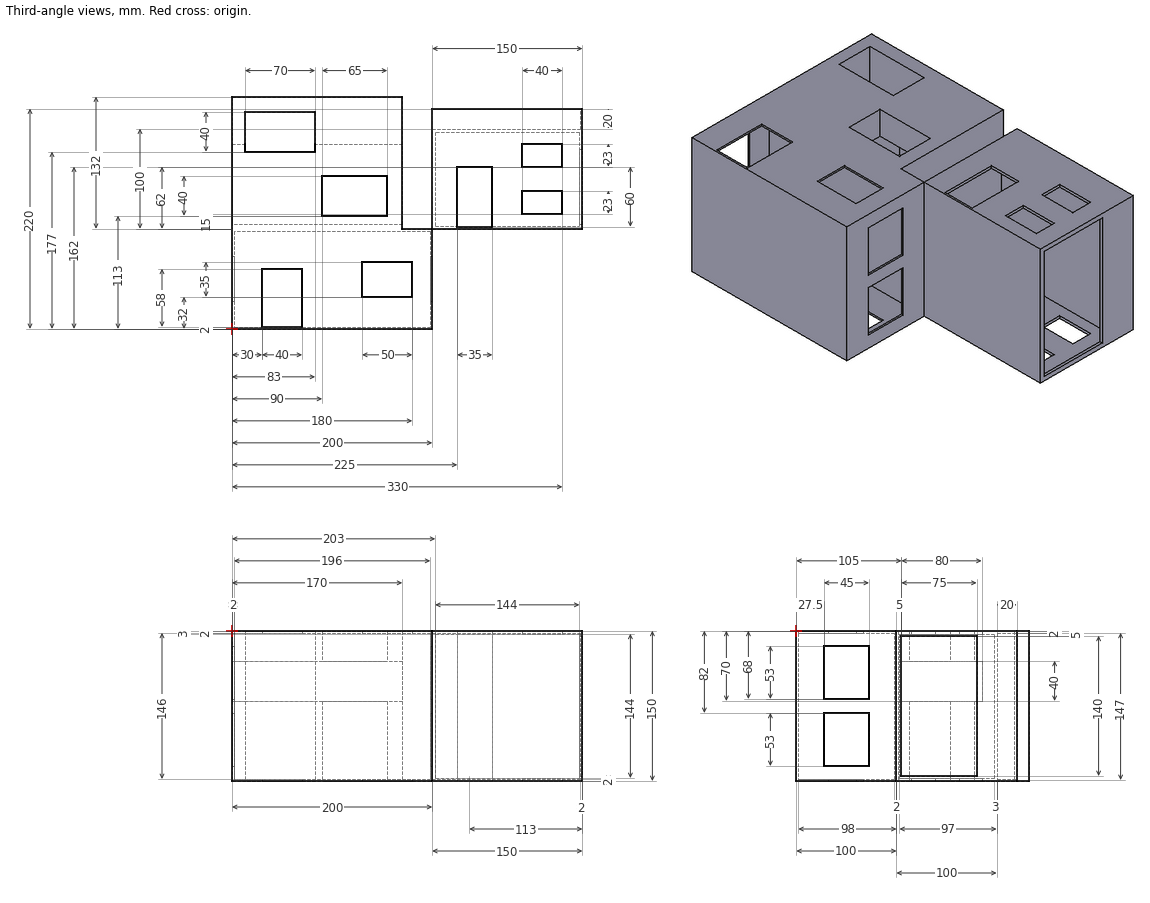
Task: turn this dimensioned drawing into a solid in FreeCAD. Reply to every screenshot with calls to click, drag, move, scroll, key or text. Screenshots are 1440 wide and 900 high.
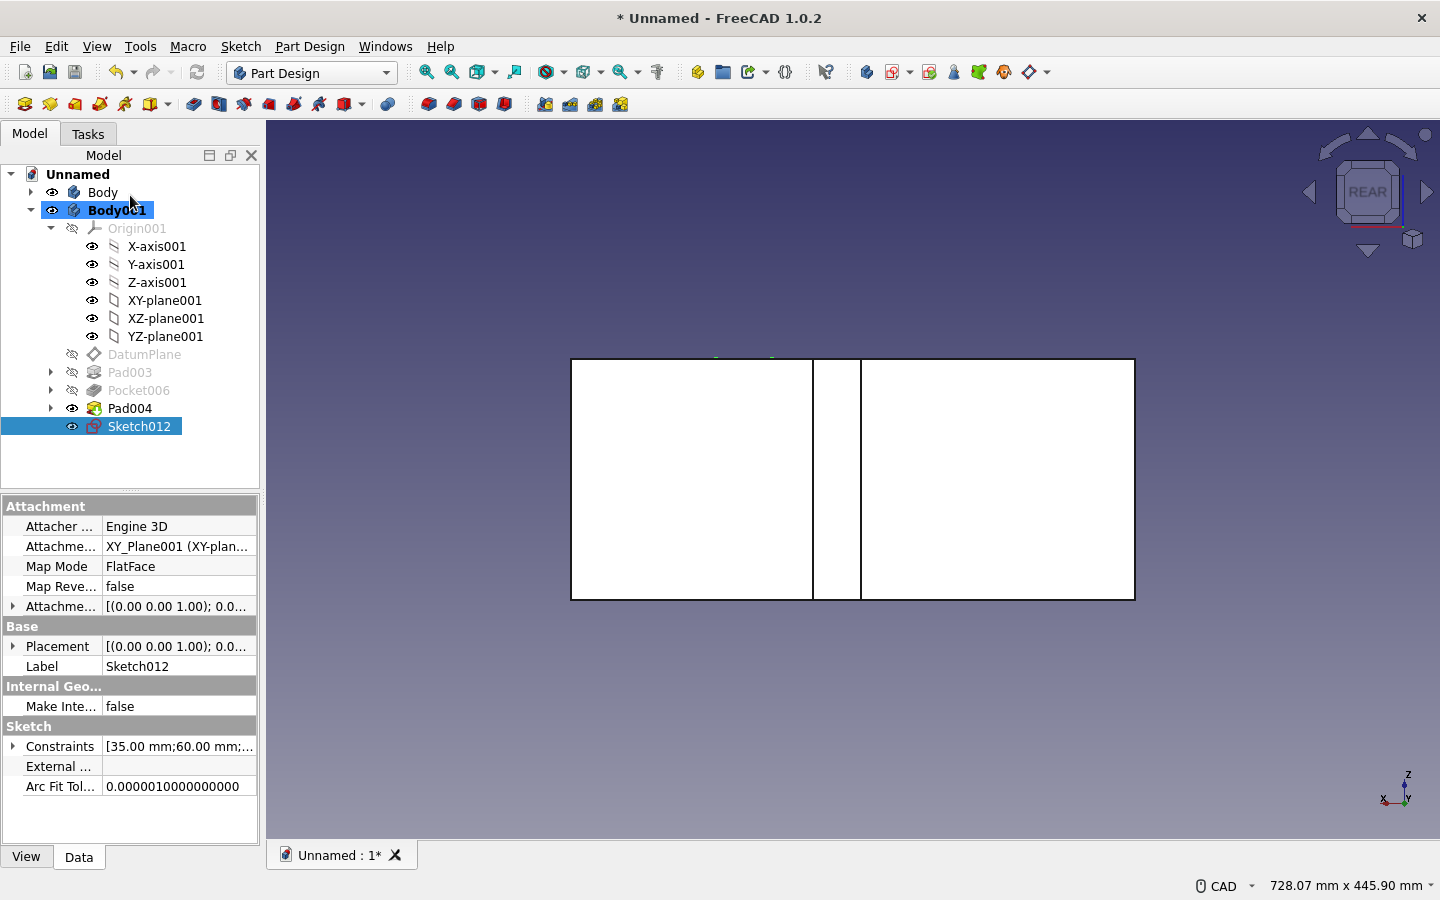
click(194, 104)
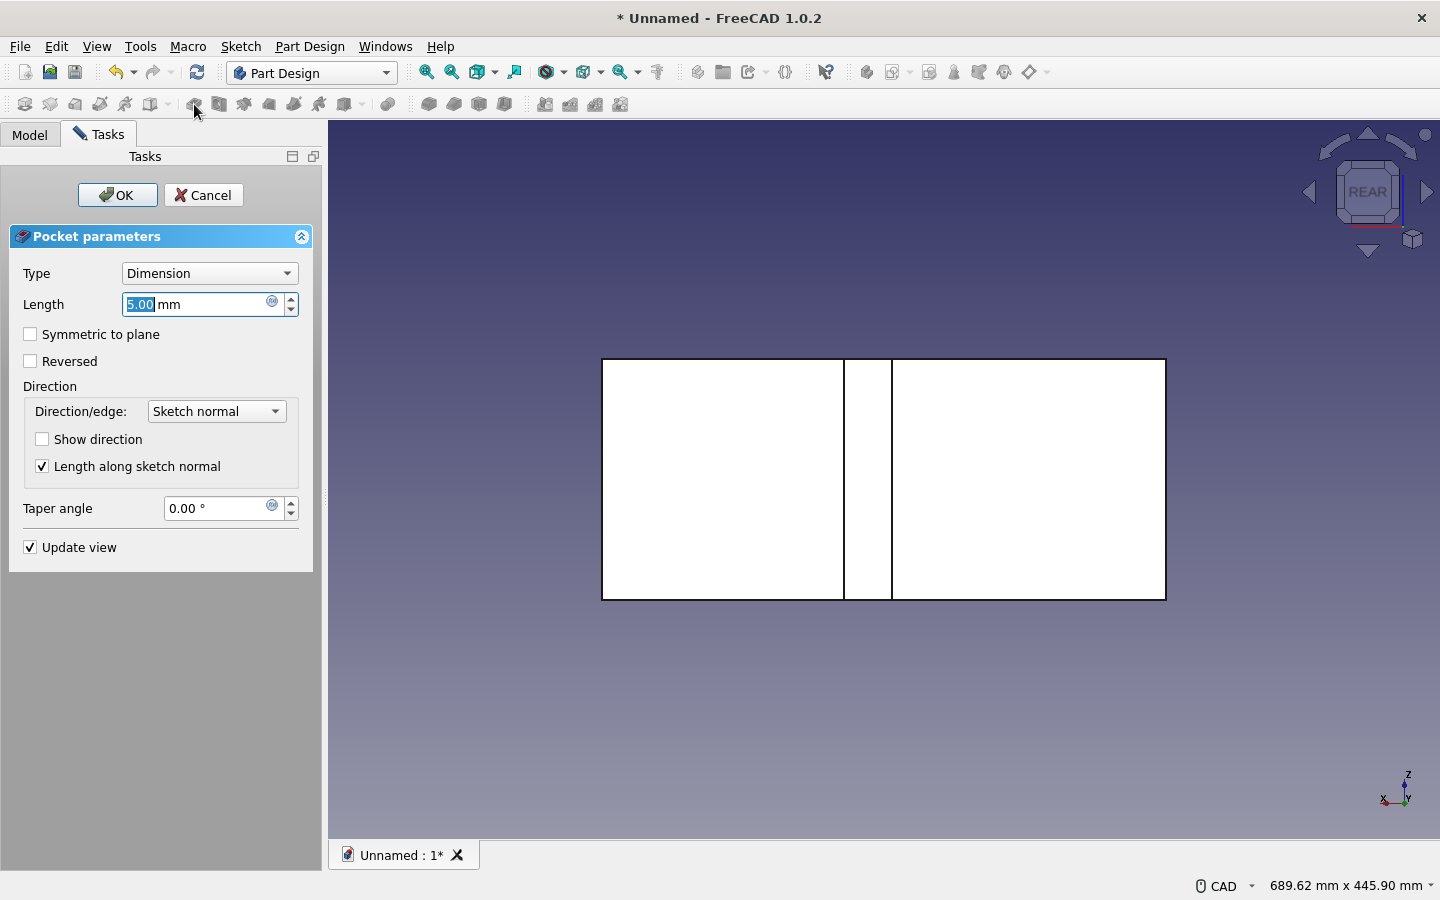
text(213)
key(Tab)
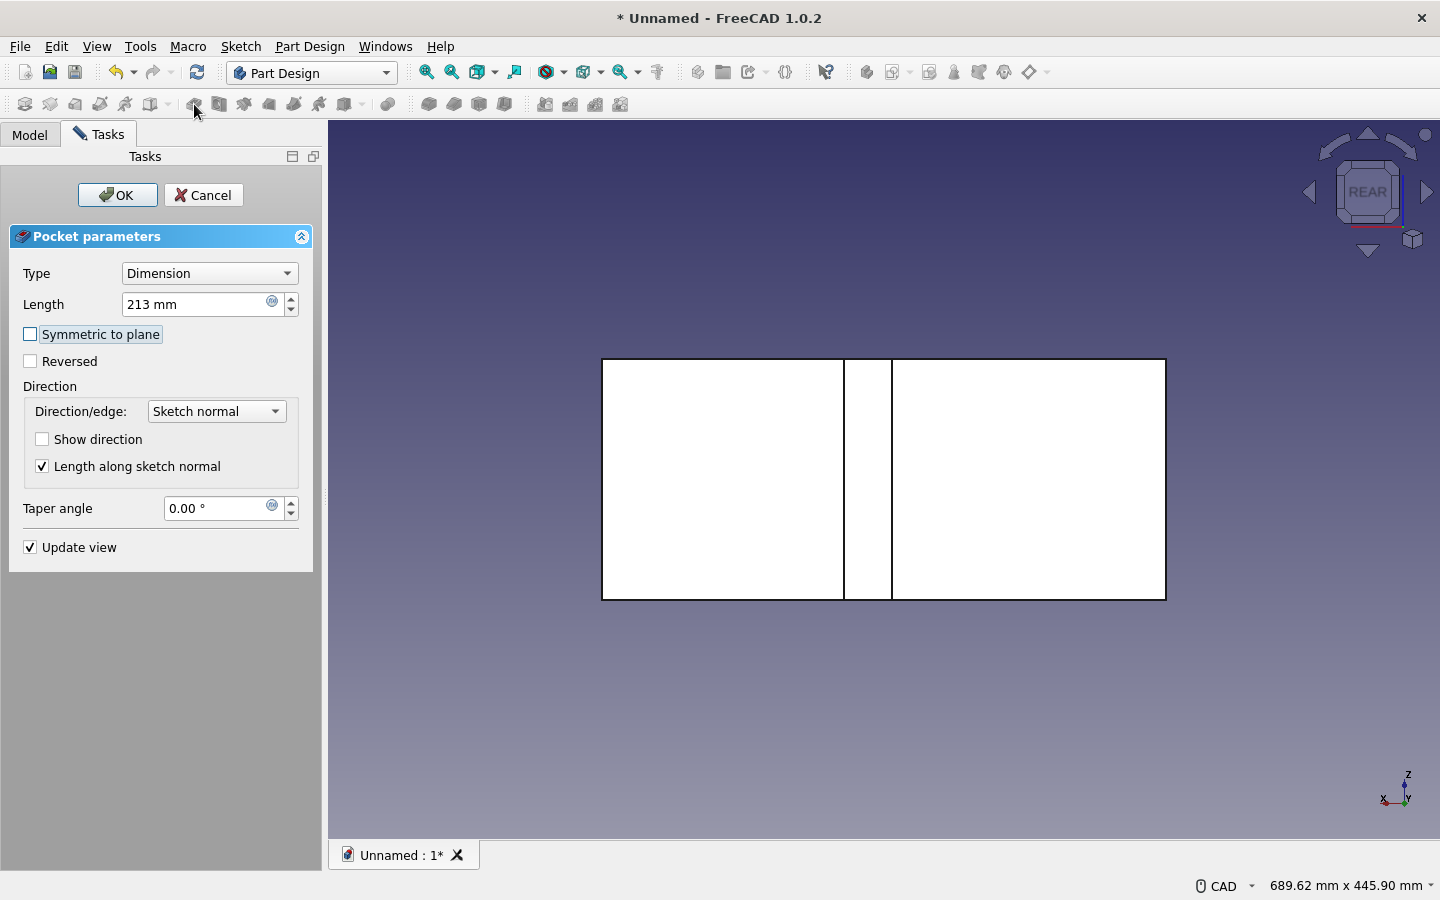
click(118, 195)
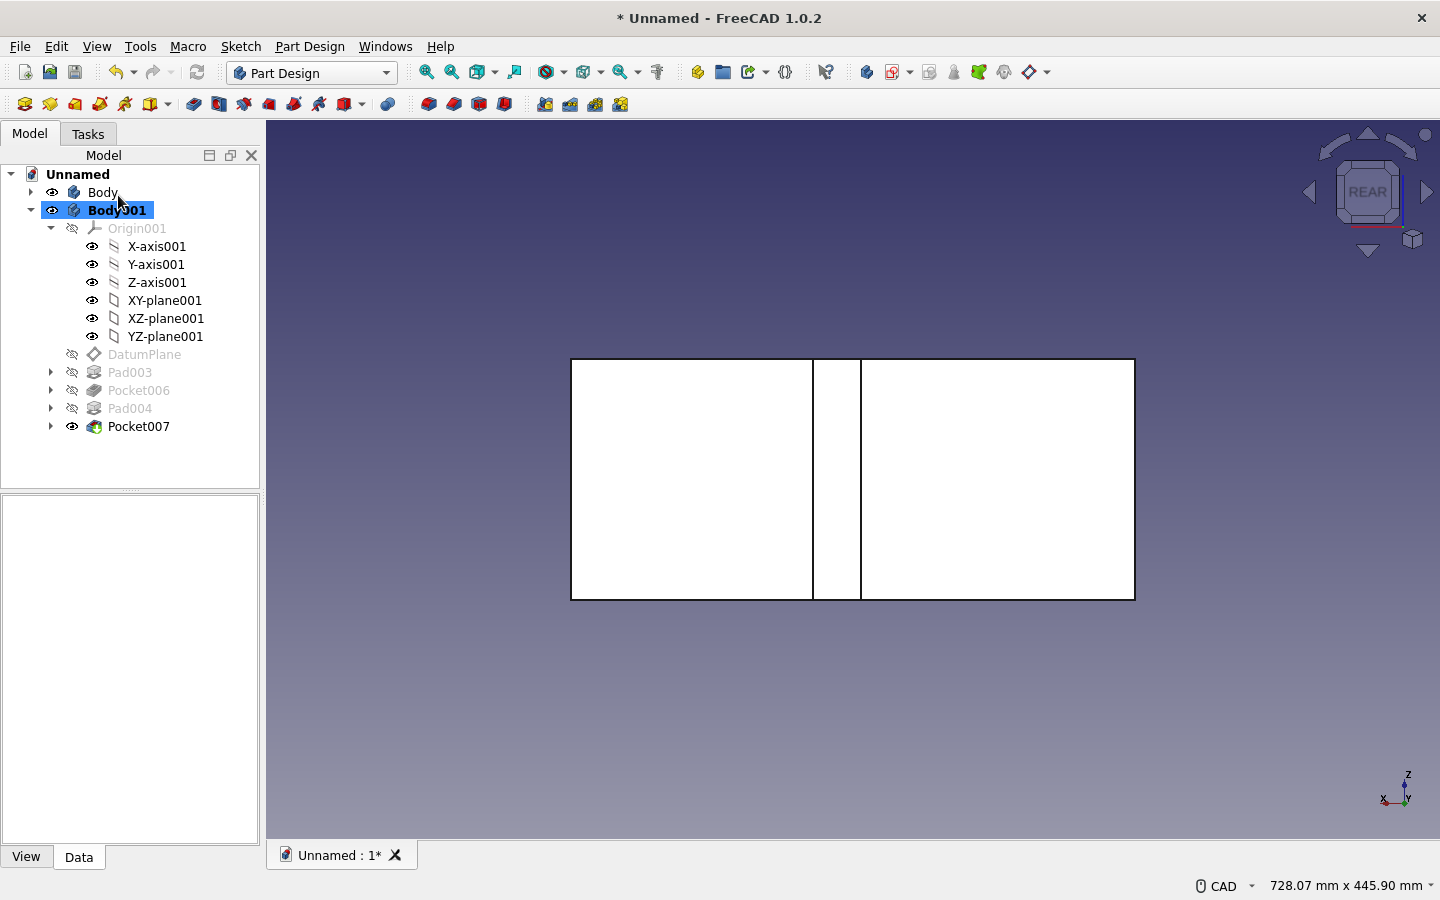
click(427, 72)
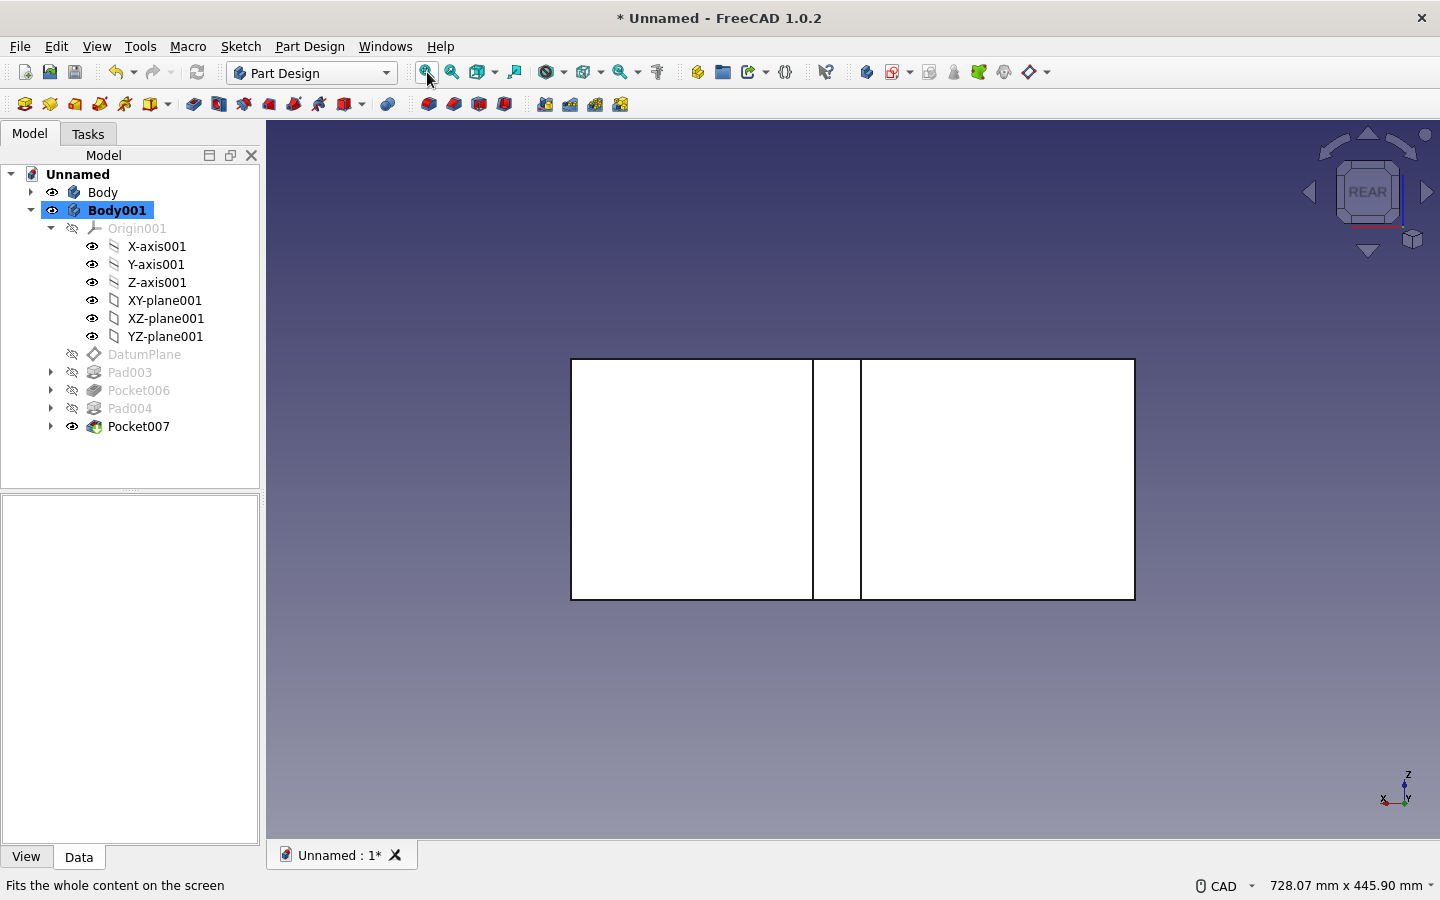
key(0)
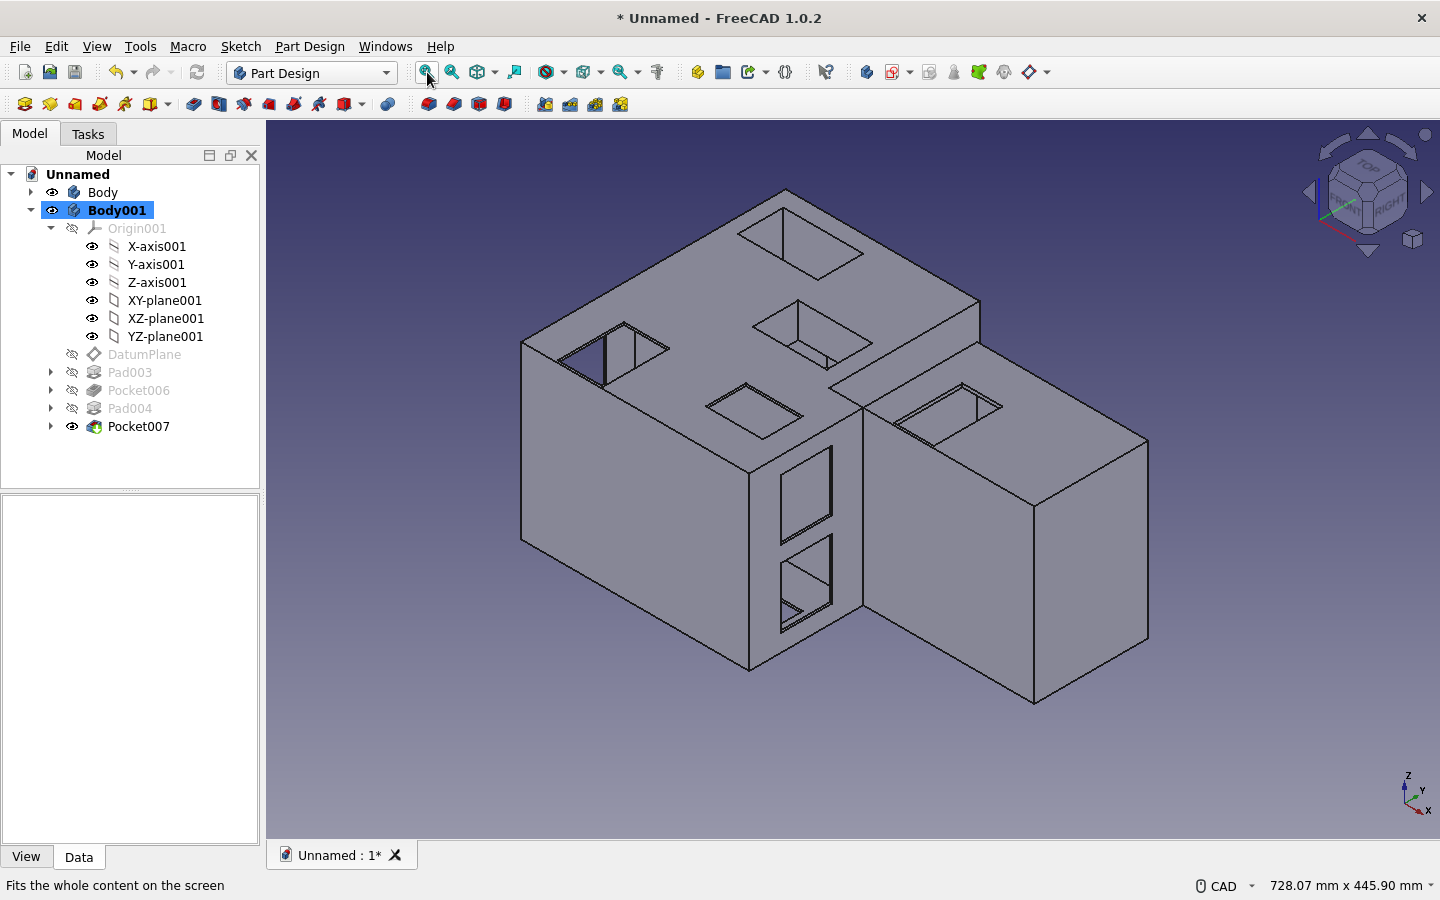
click(1030, 437)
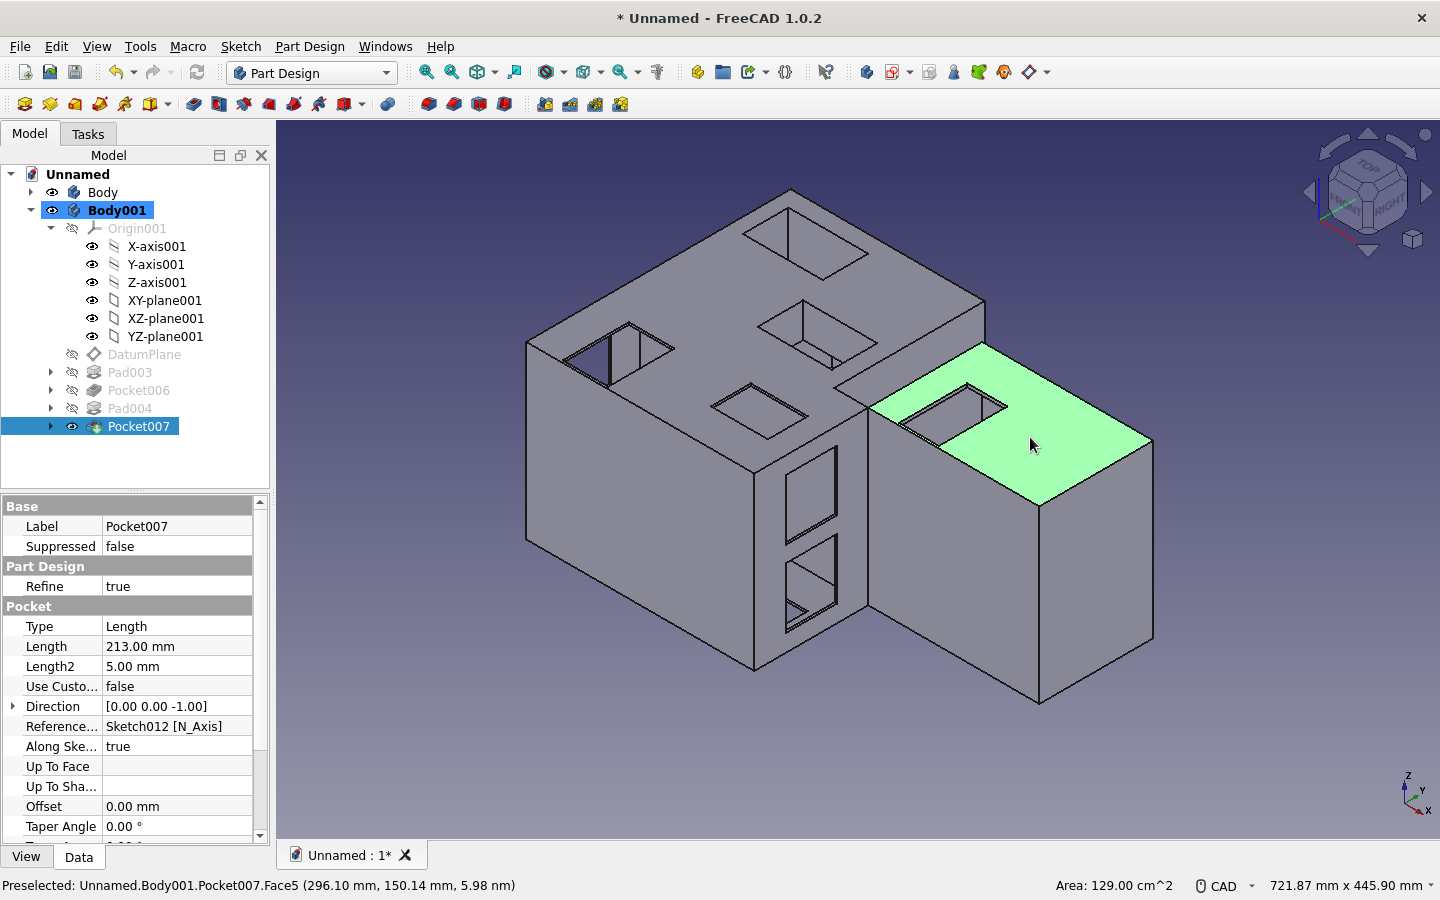
click(892, 72)